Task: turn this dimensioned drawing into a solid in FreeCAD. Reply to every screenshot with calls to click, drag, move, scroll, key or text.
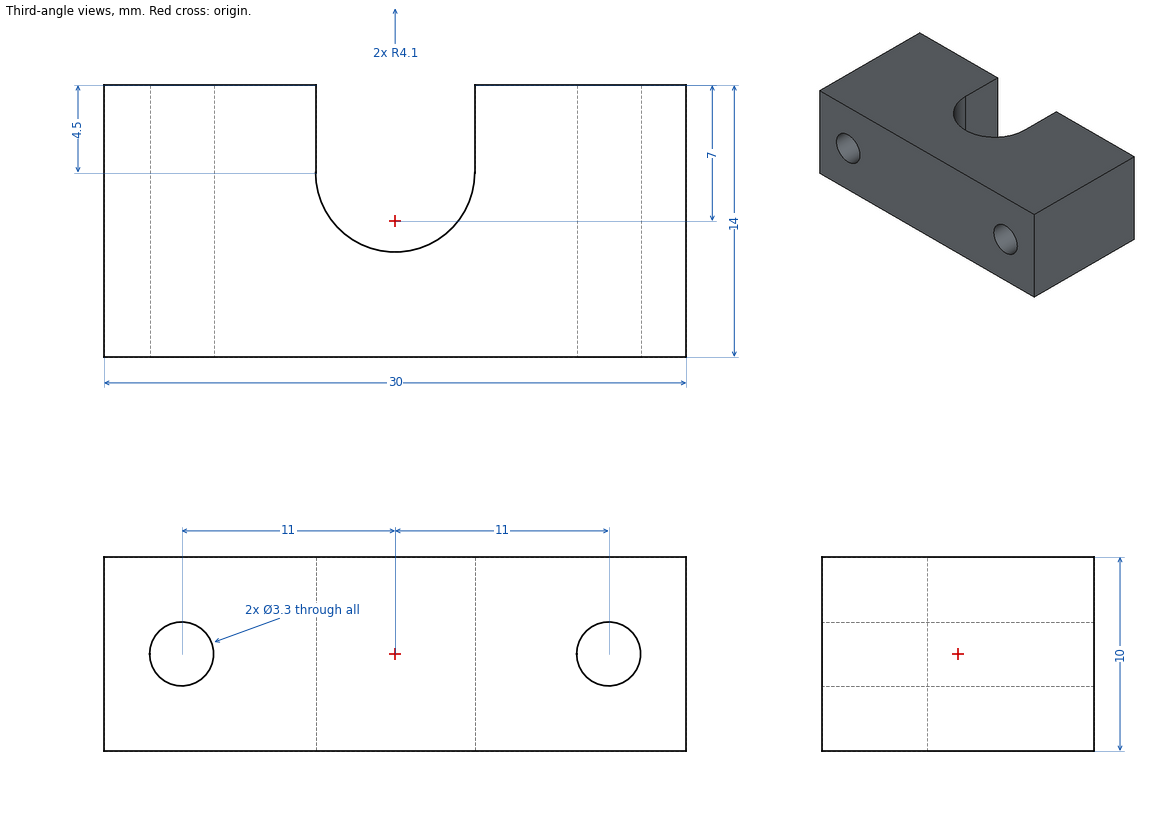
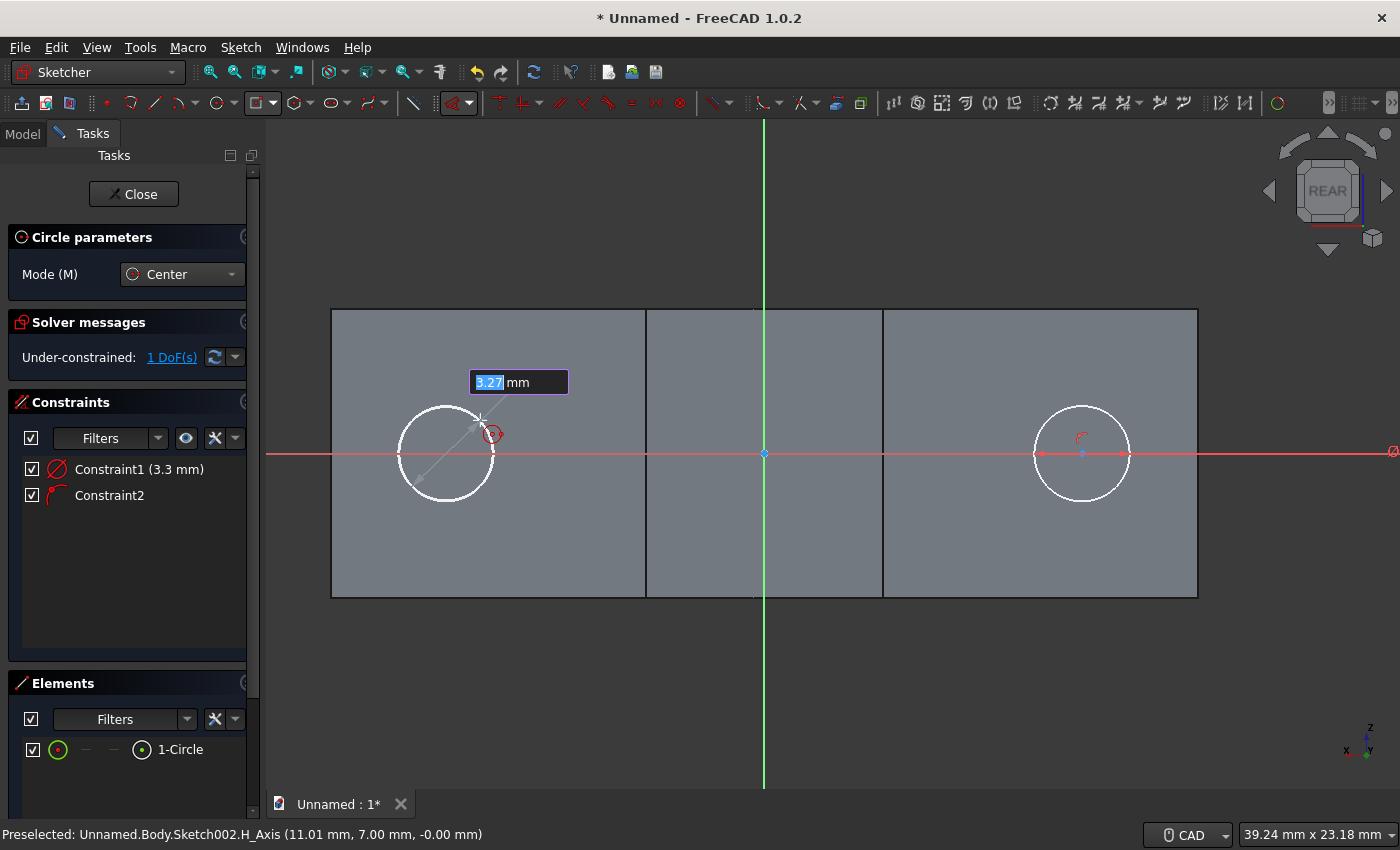
text(3.3)
key(Return)
key(Escape)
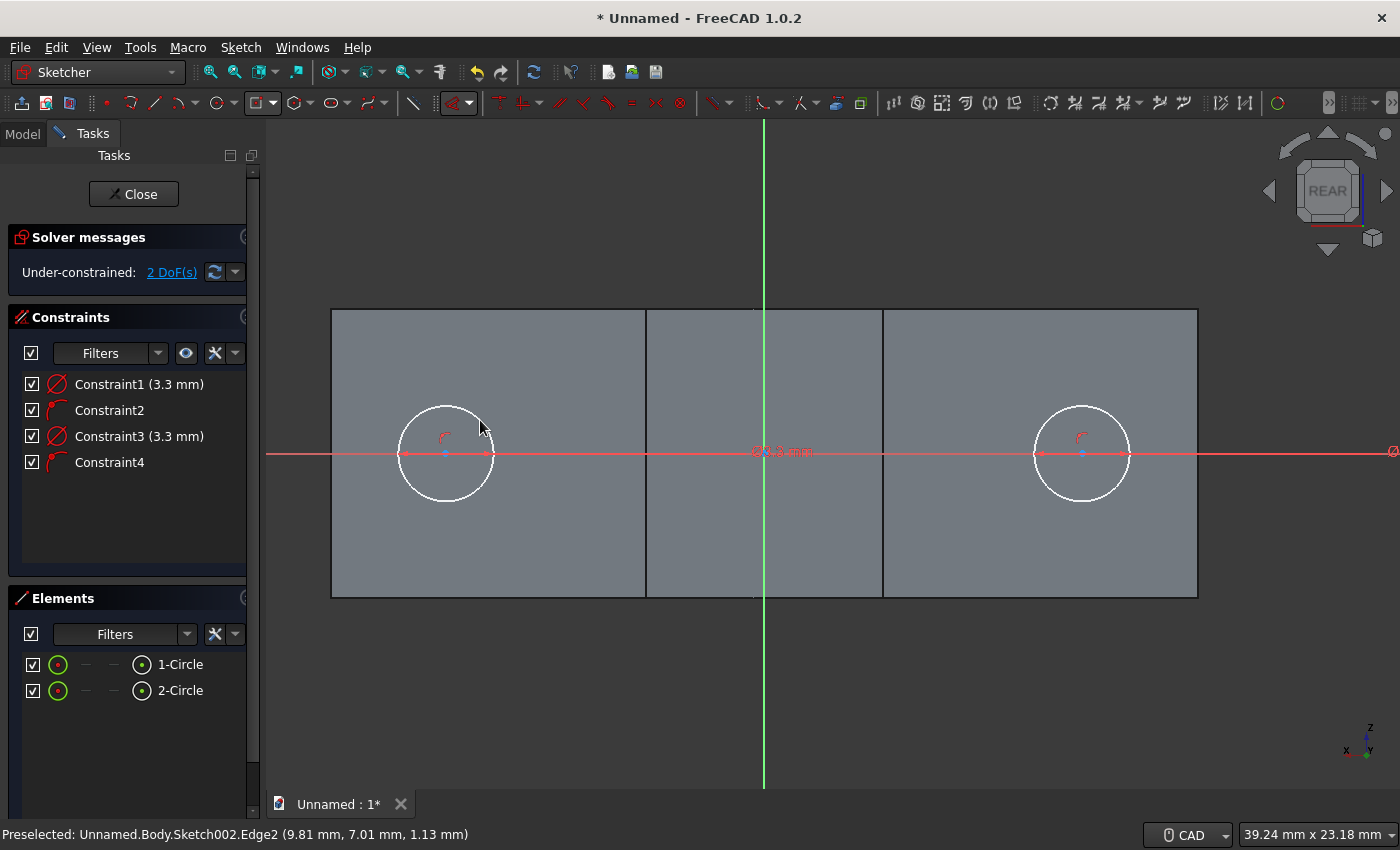
click(1082, 454)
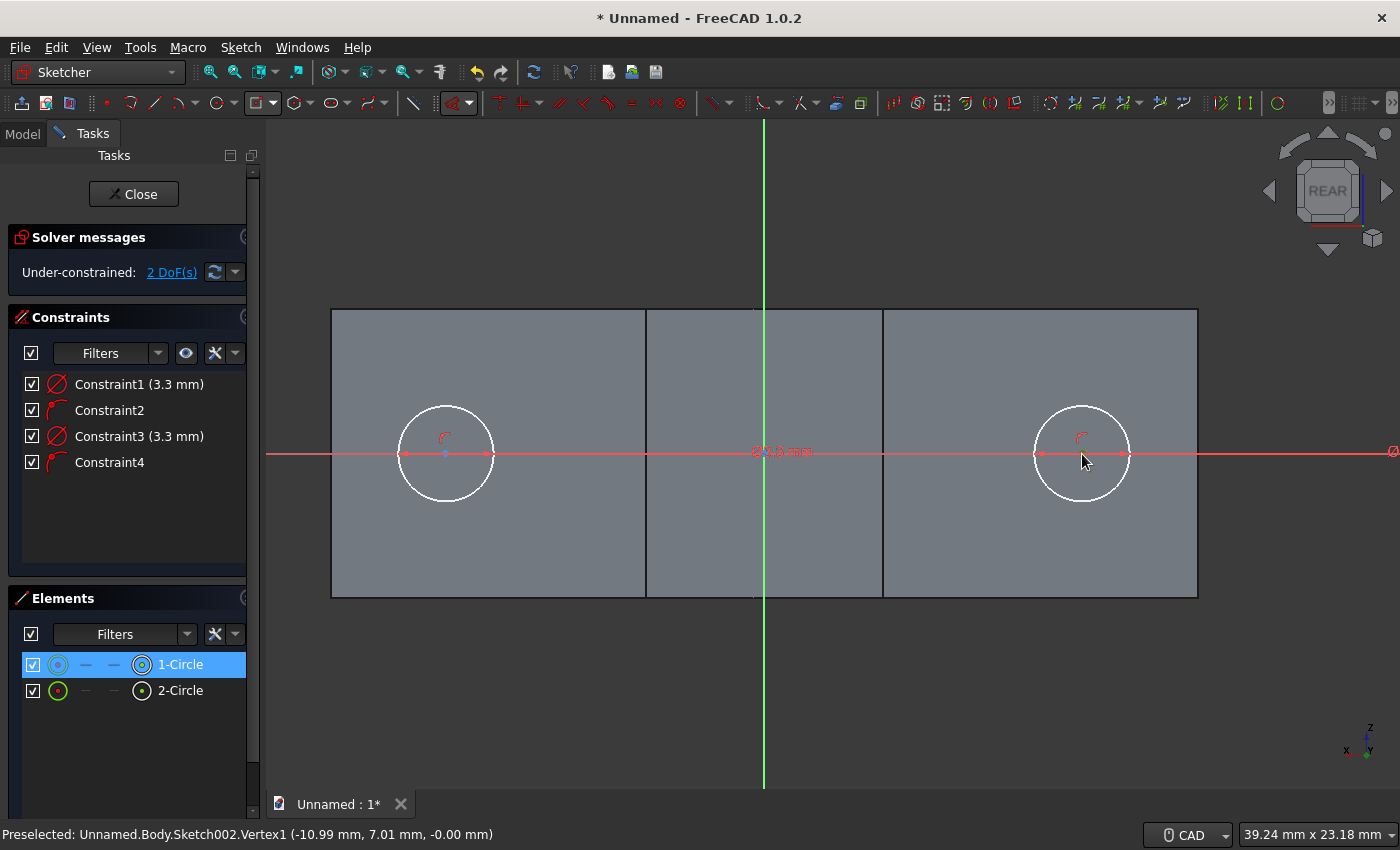
key(l)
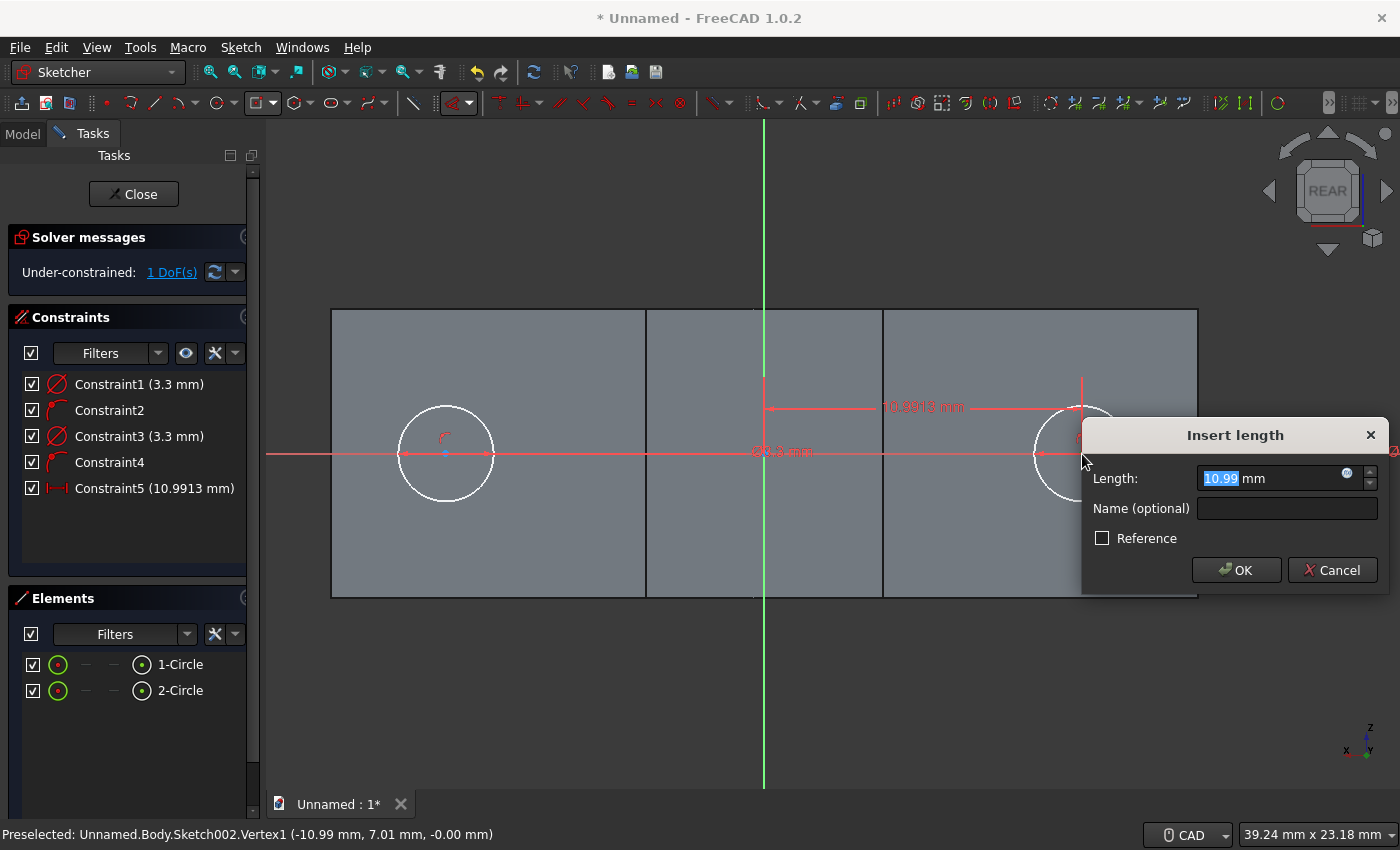
text(11)
key(Return)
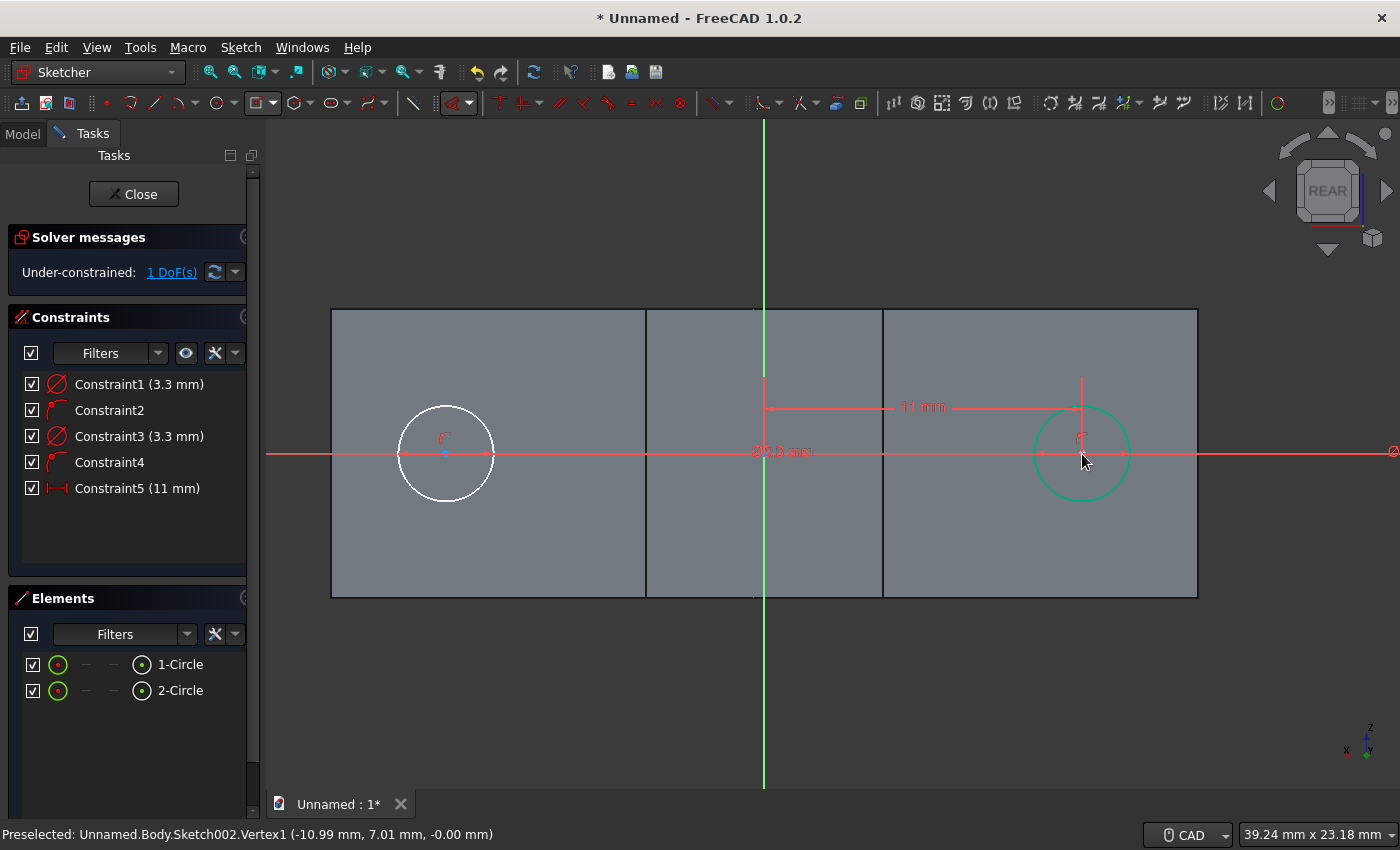
click(446, 454)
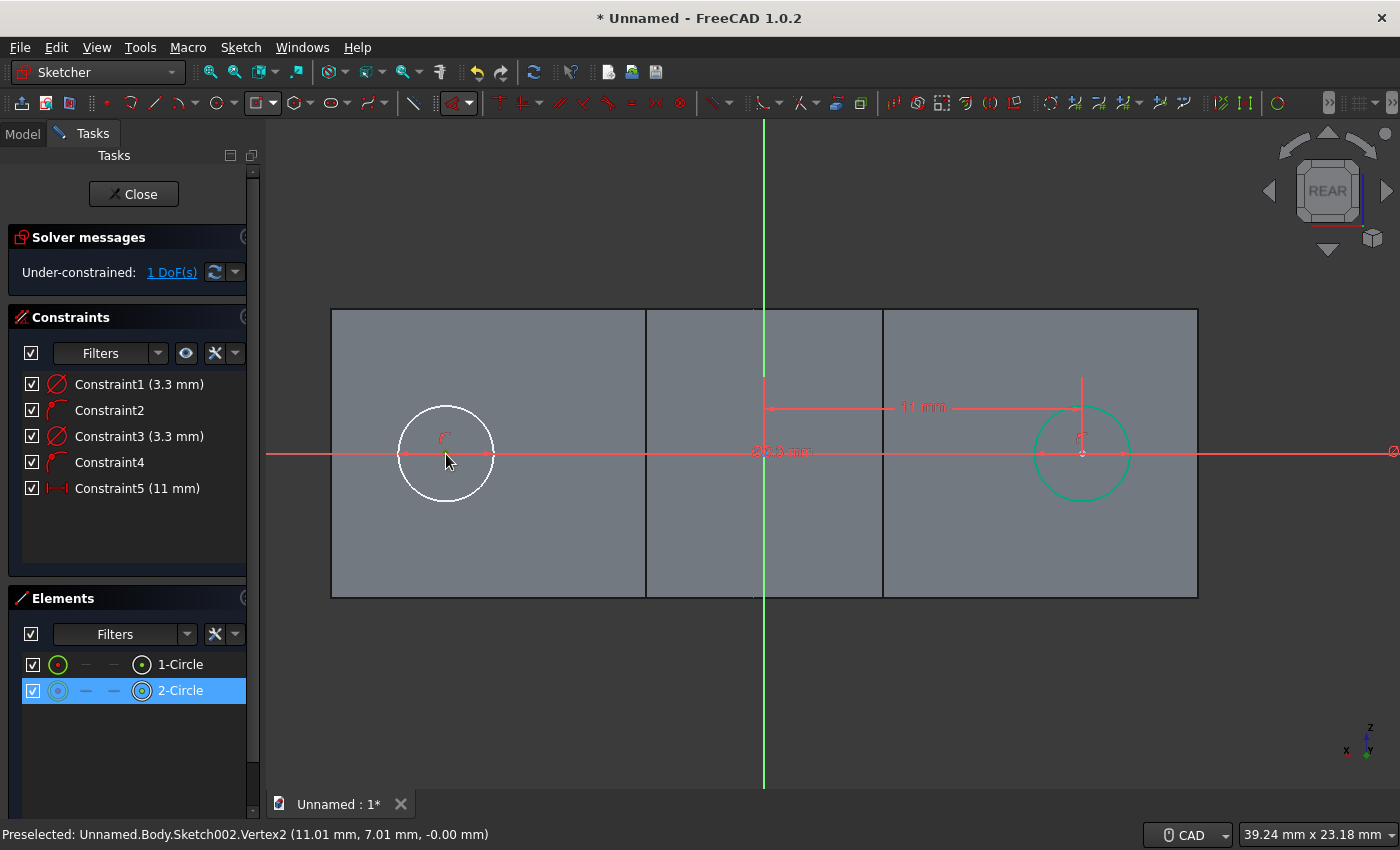
key(l)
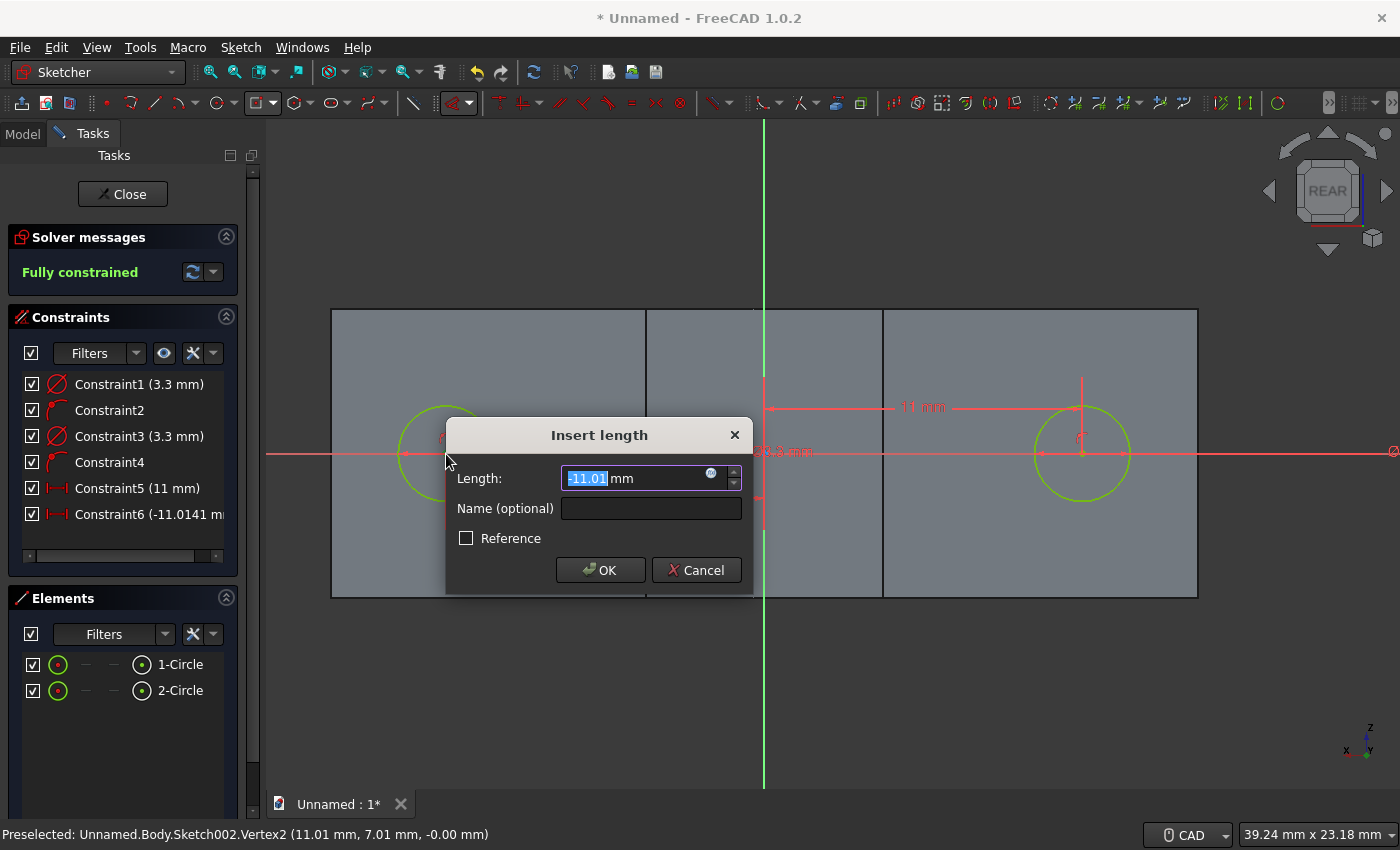
text(-11)
key(Return)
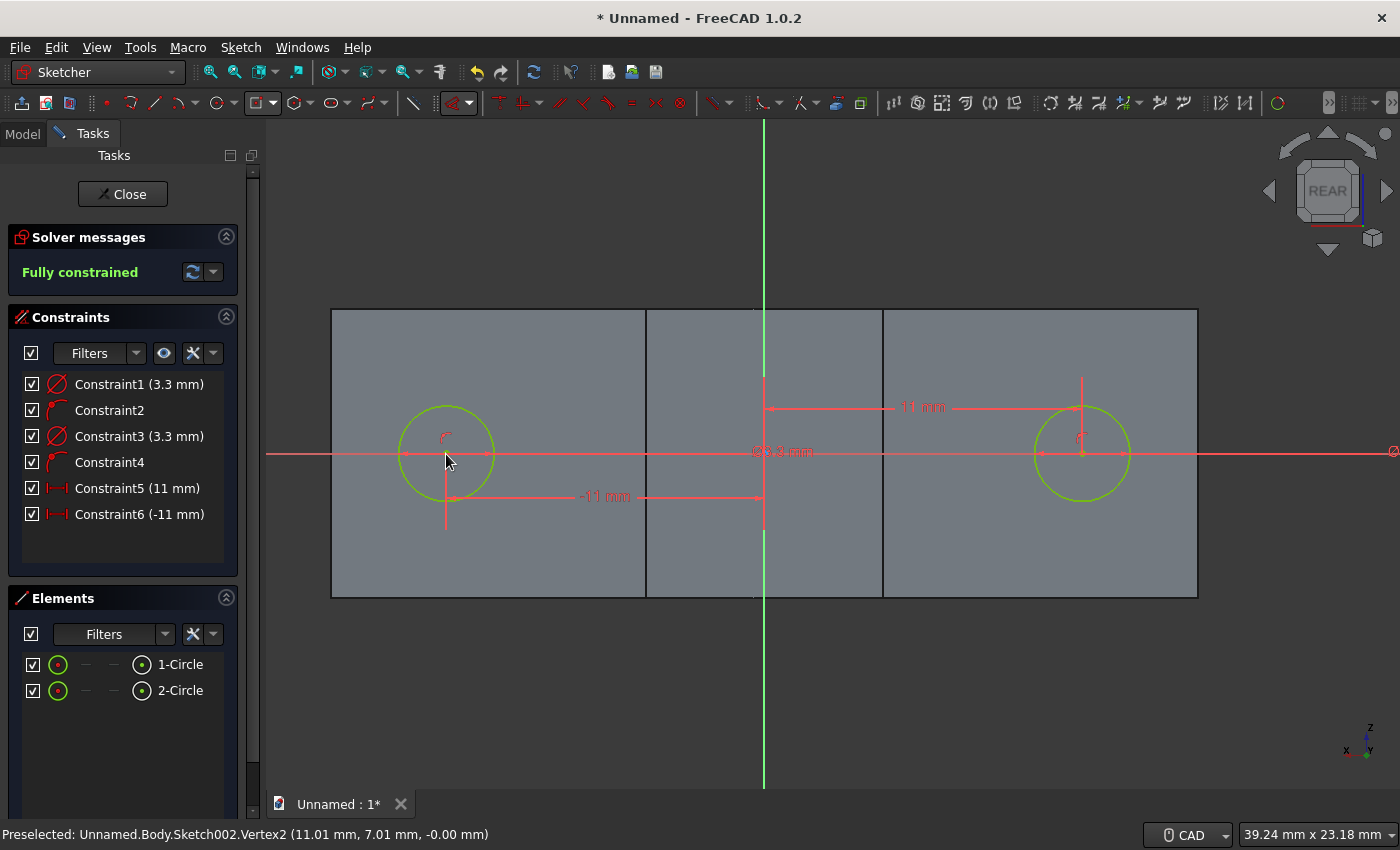
click(123, 194)